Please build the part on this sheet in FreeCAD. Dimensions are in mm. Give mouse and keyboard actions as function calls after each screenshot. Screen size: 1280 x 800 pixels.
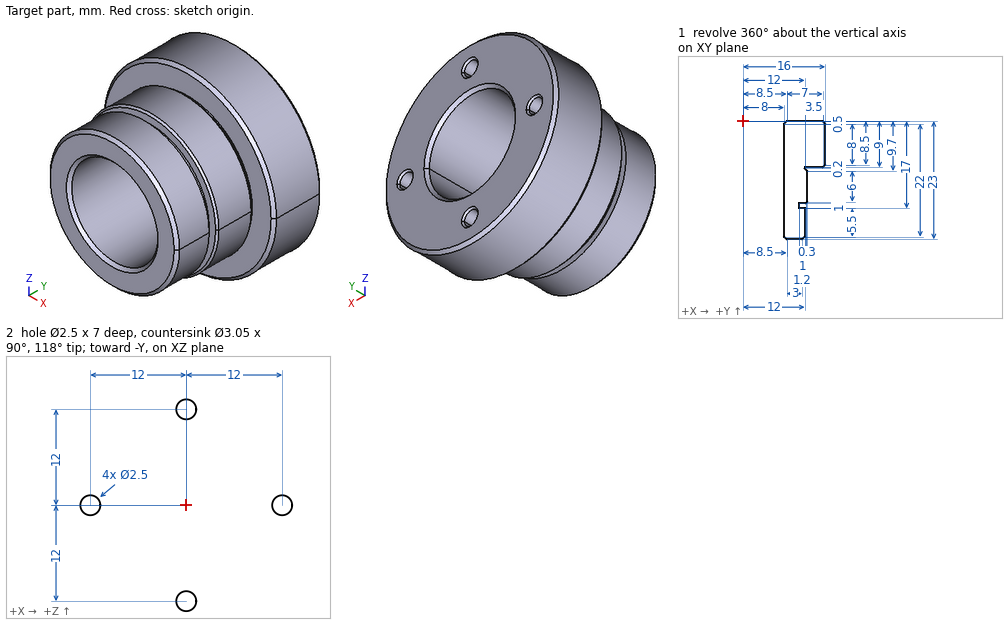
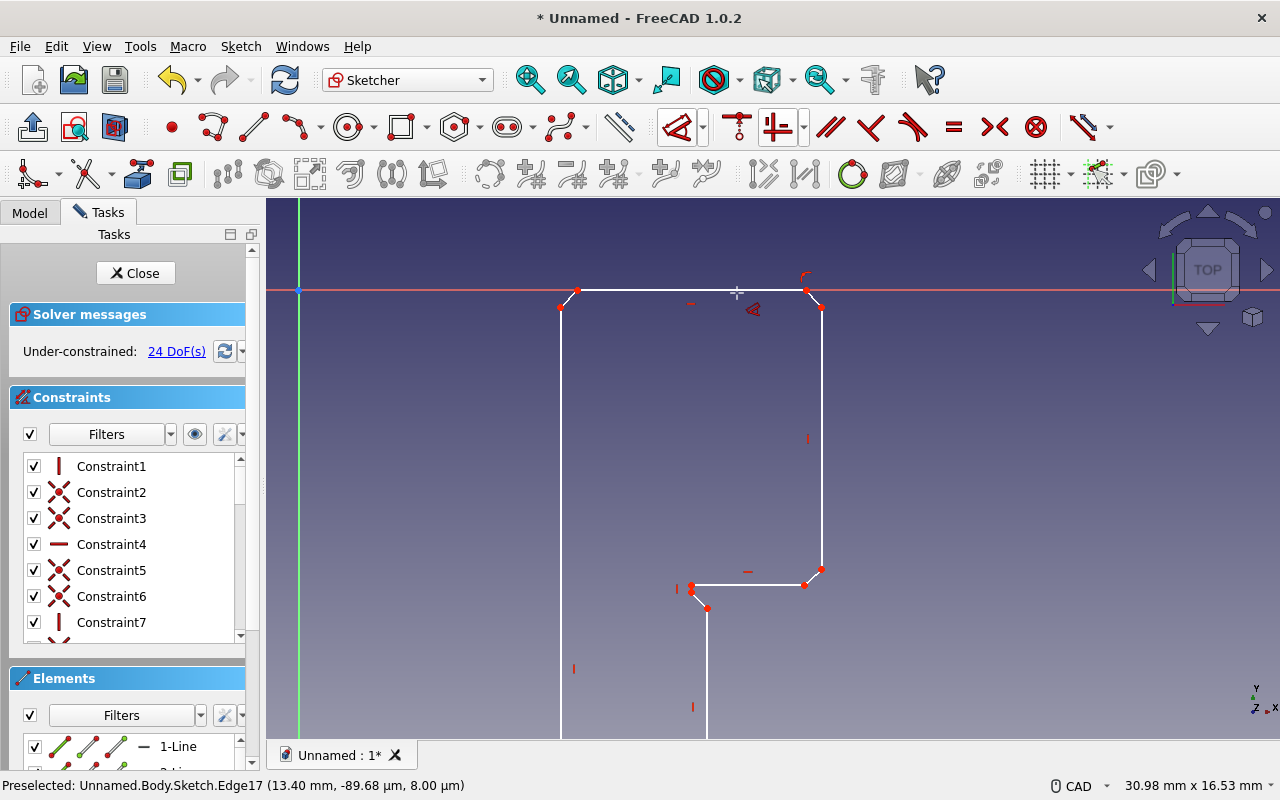
scroll(822, 307, down, 4)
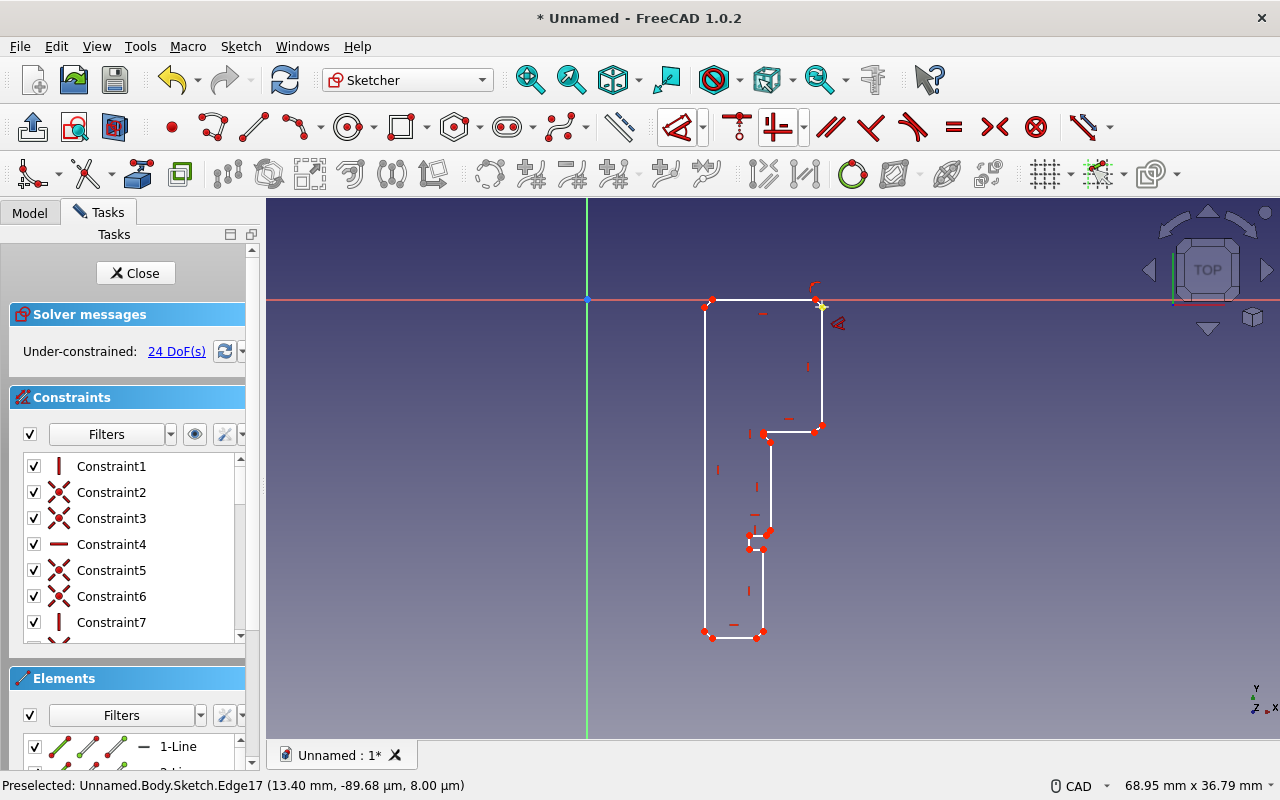
click(726, 638)
click(734, 672)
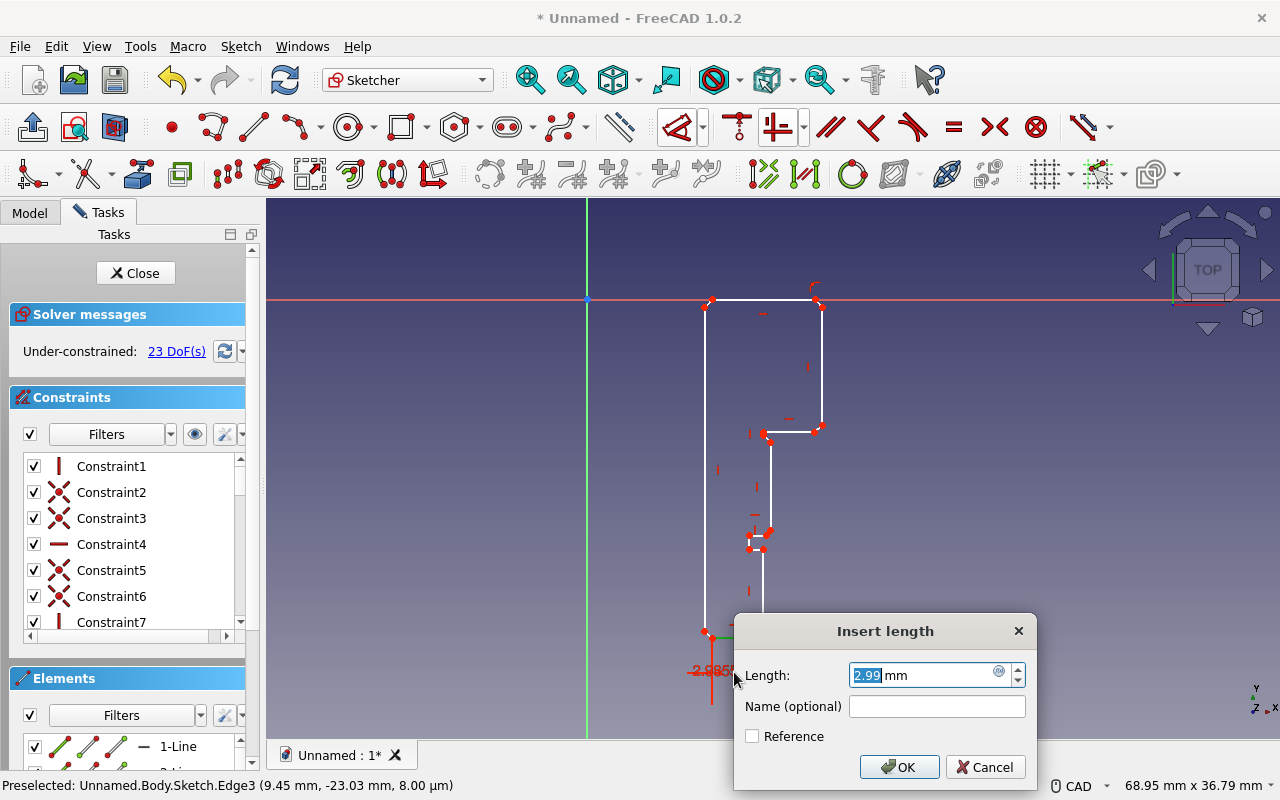
text(3)
key(Return)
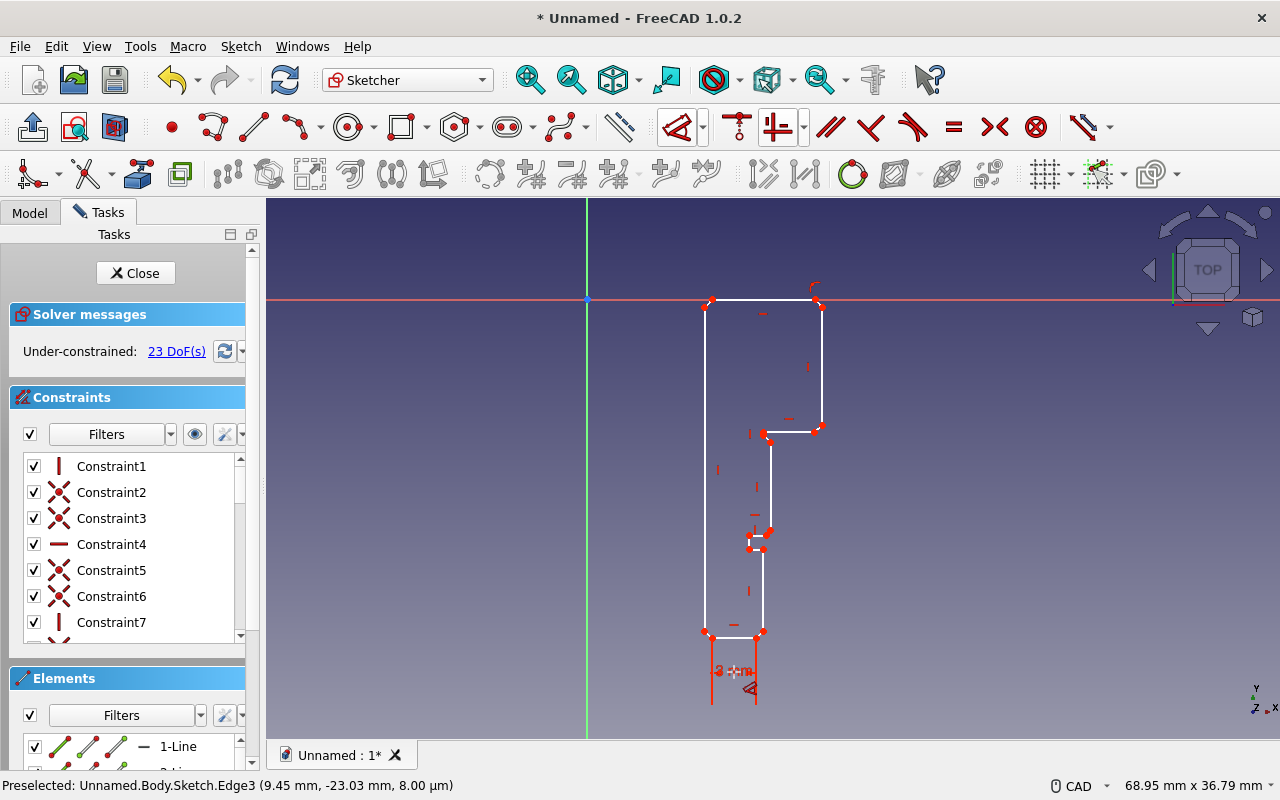
scroll(756, 550, up, 5)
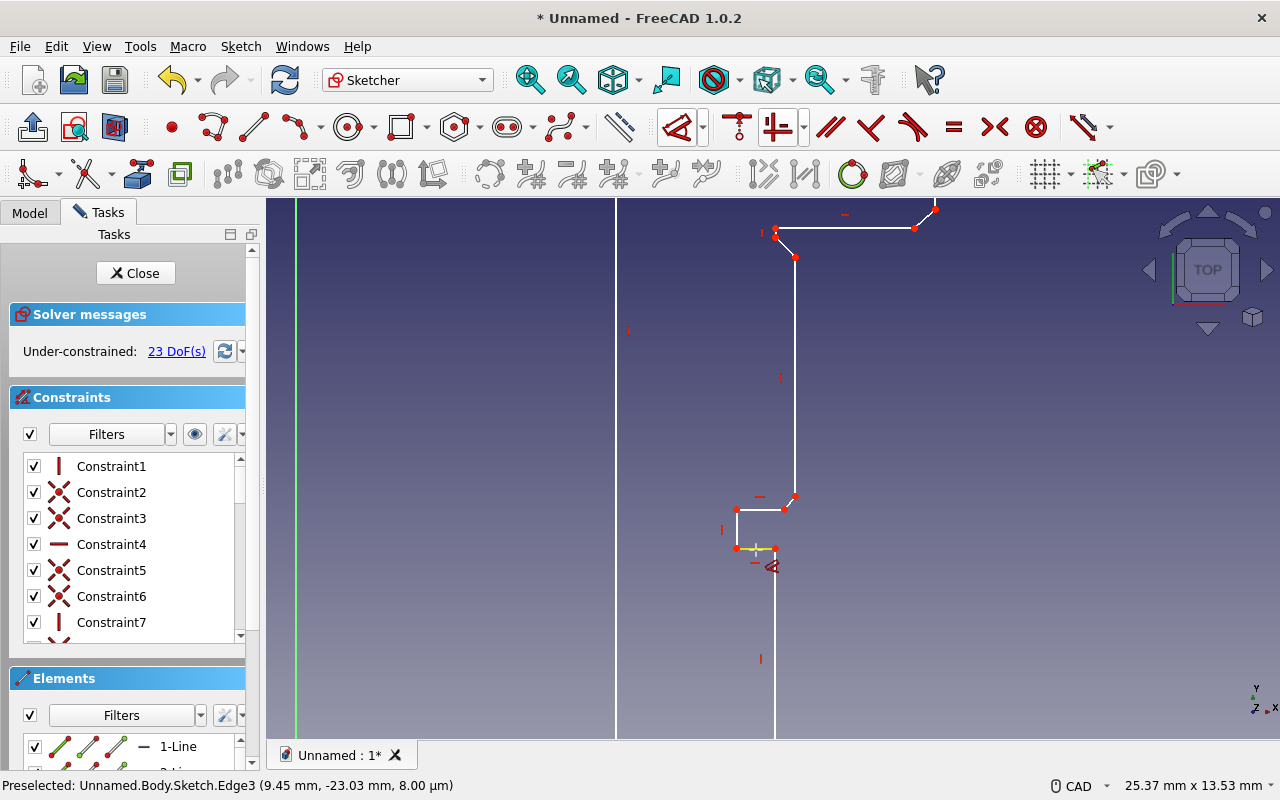
click(756, 549)
click(756, 583)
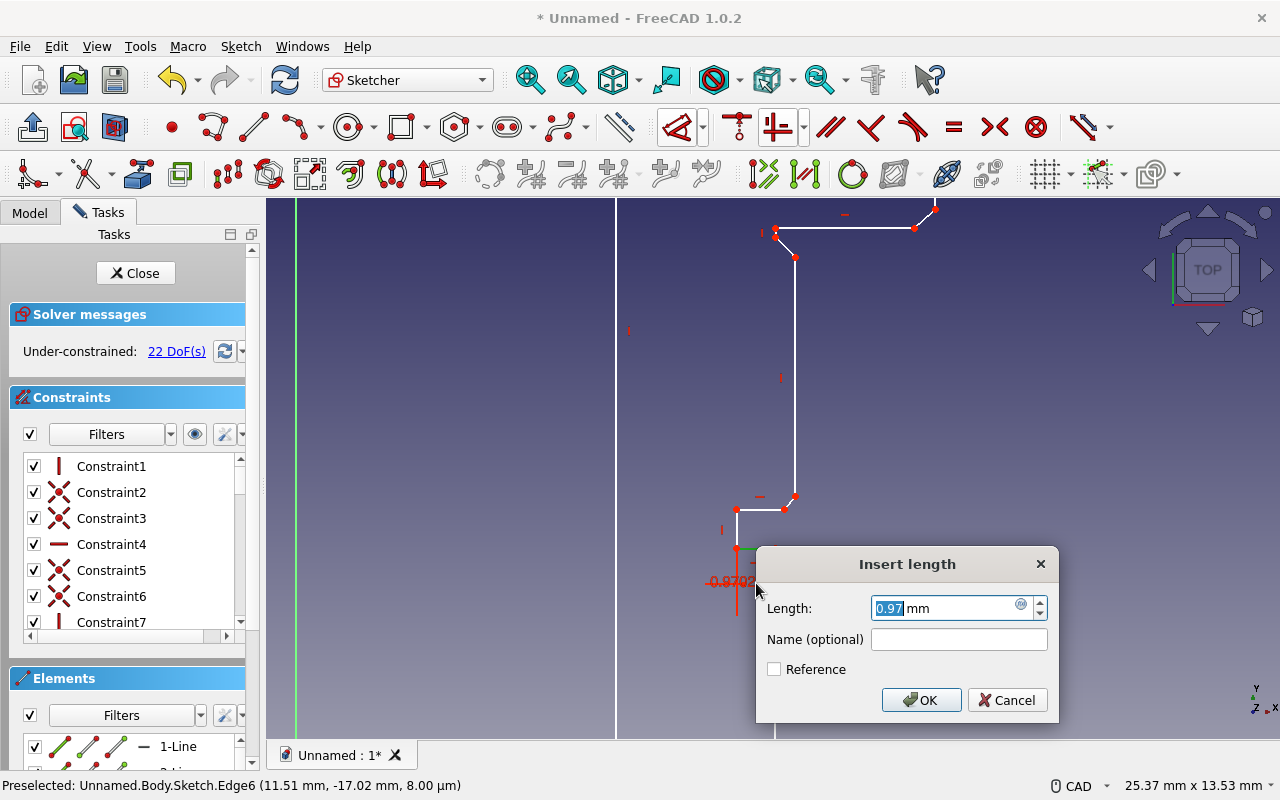
text(1)
key(Return)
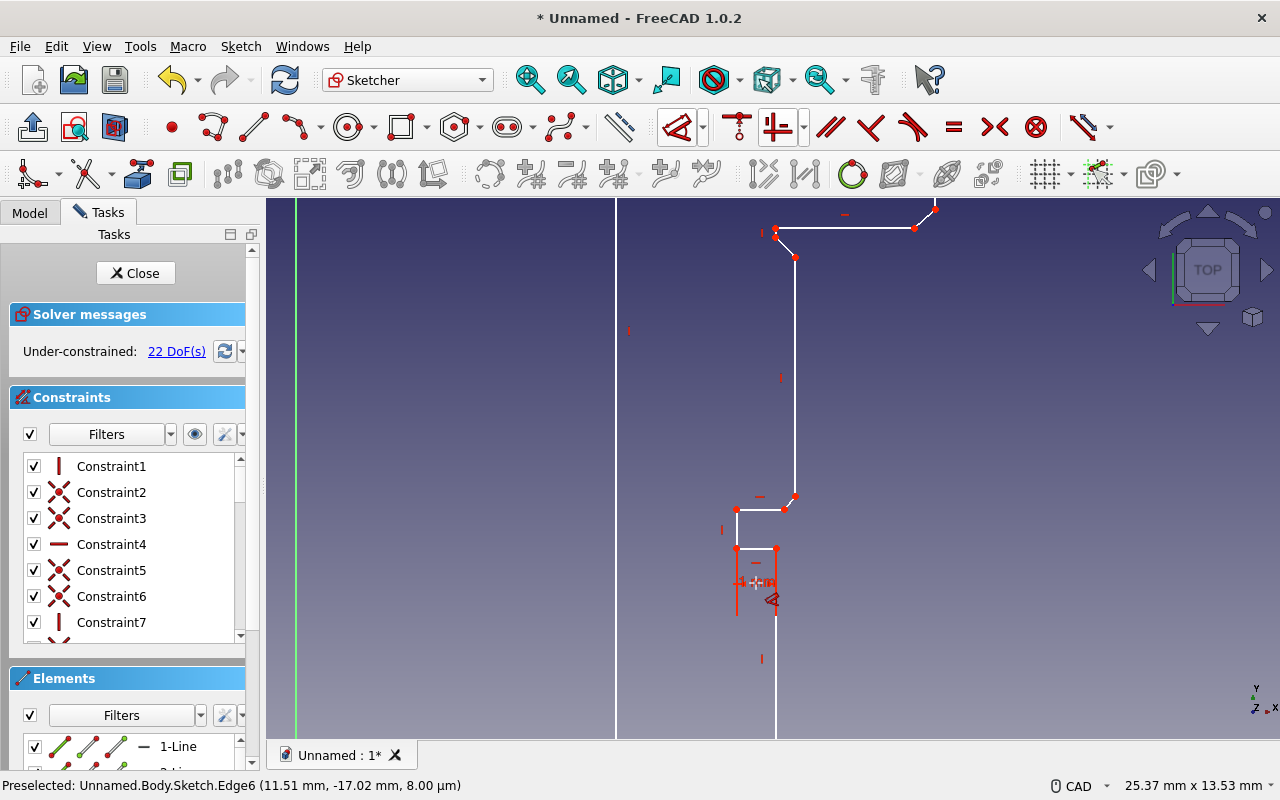
click(737, 537)
click(771, 529)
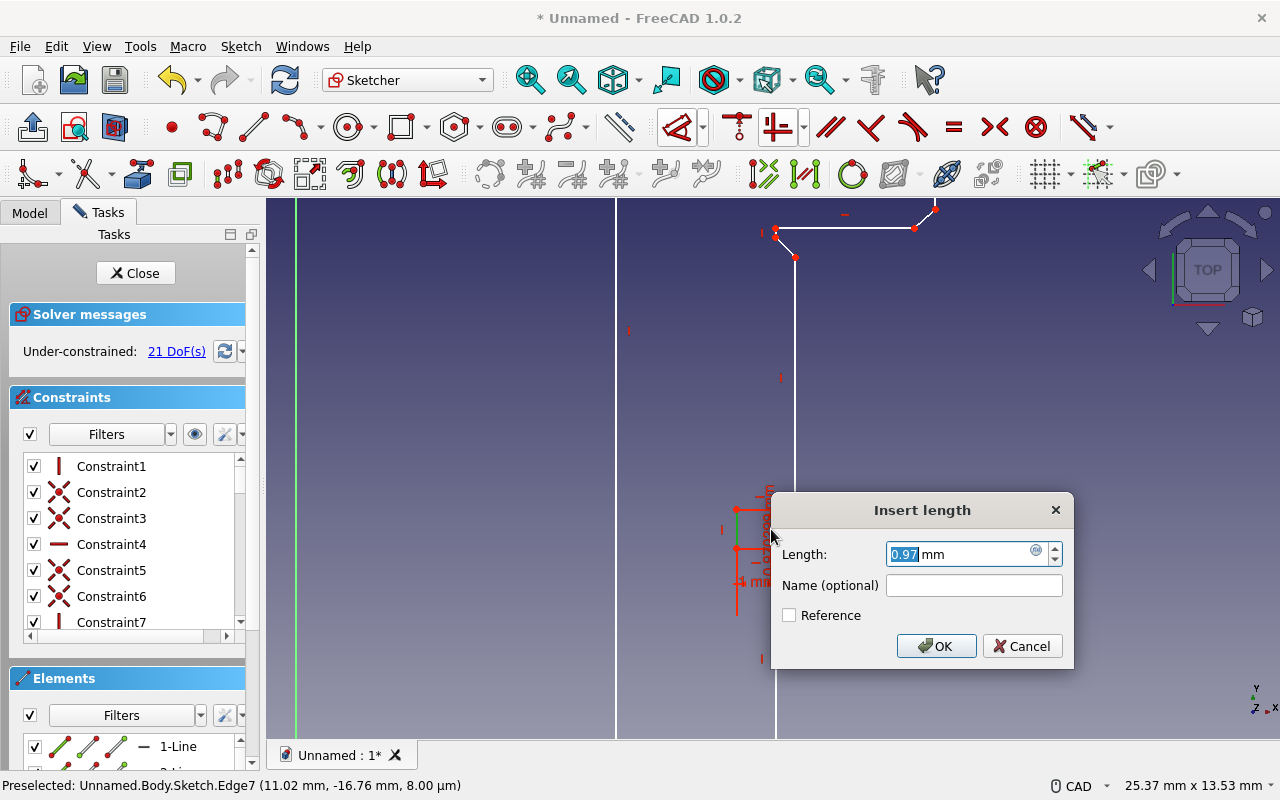
text(1)
key(Return)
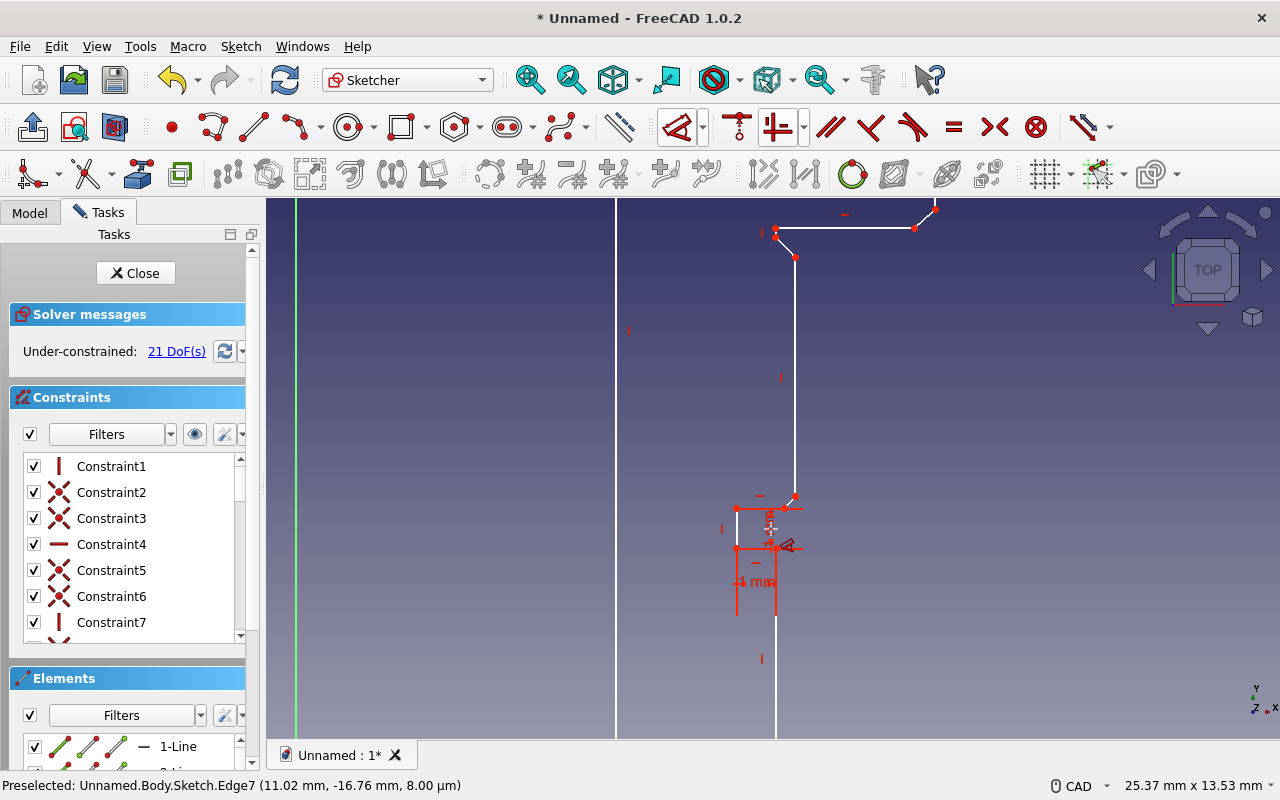
click(795, 425)
click(829, 377)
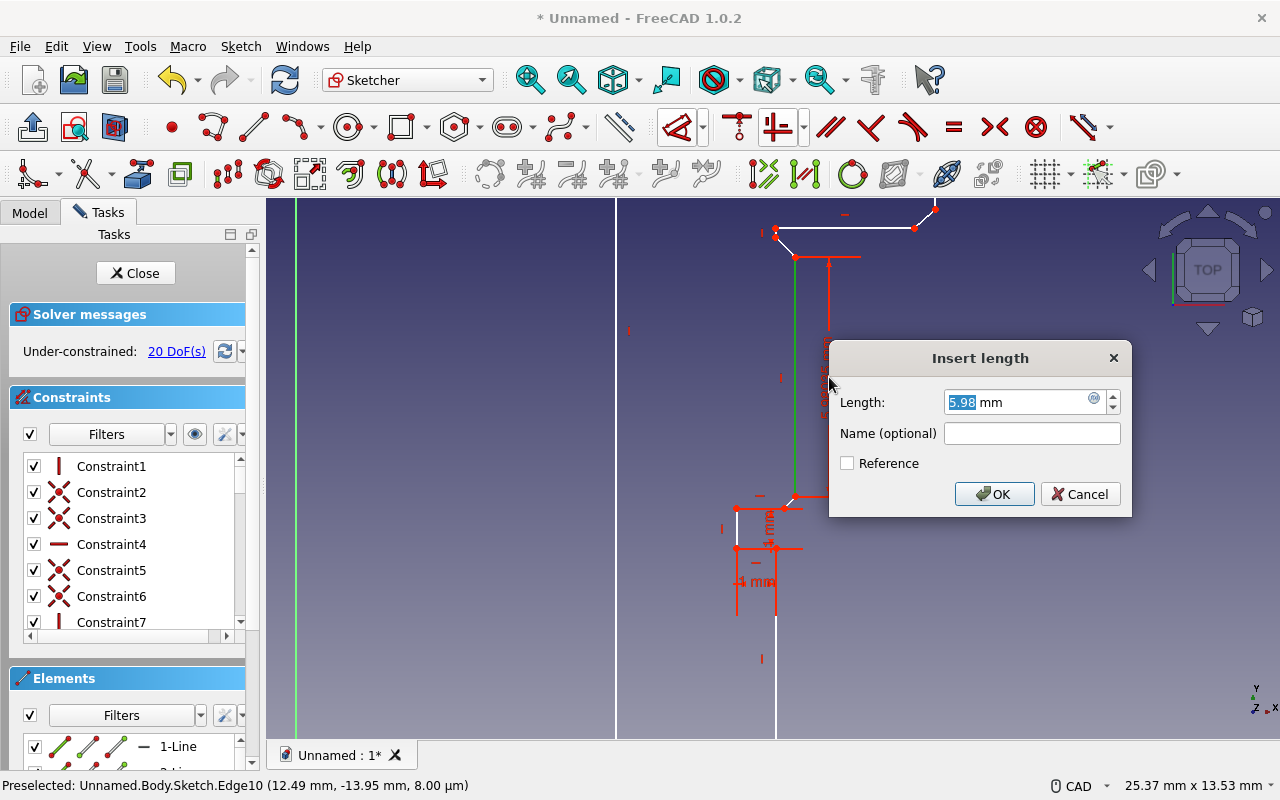
text(6)
key(Return)